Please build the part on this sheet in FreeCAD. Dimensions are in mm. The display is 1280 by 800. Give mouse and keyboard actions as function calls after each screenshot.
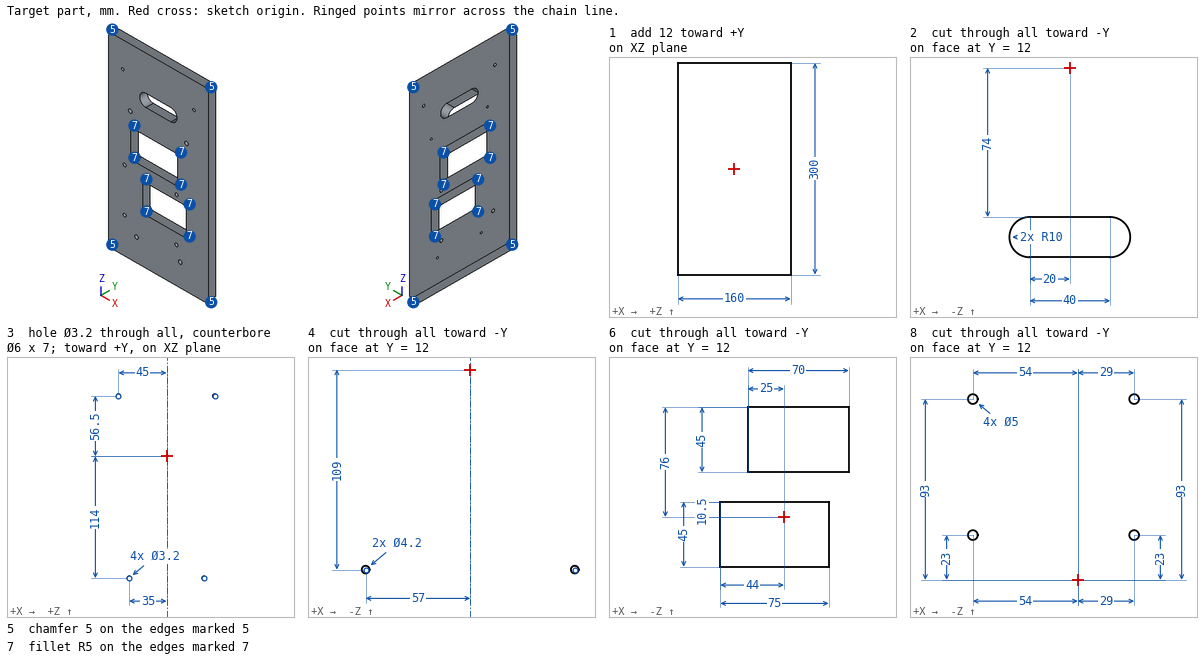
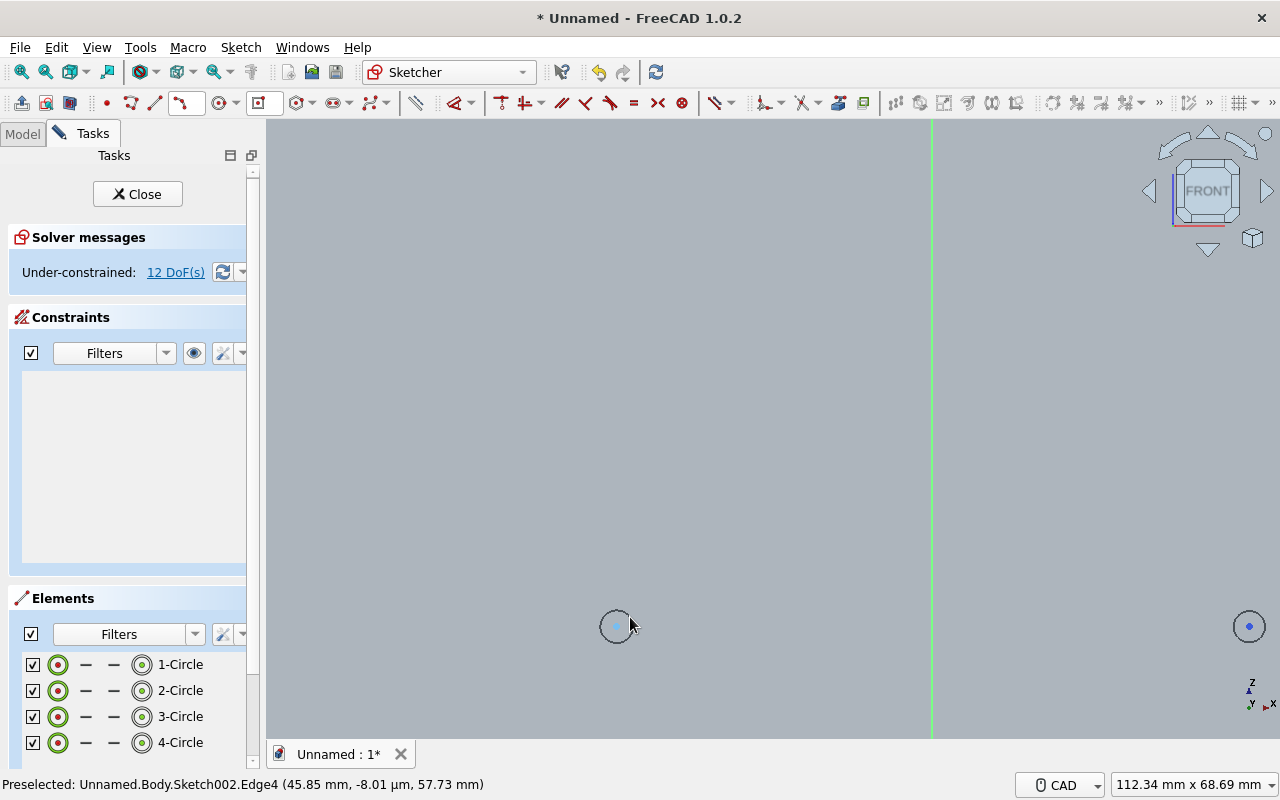
click(628, 615)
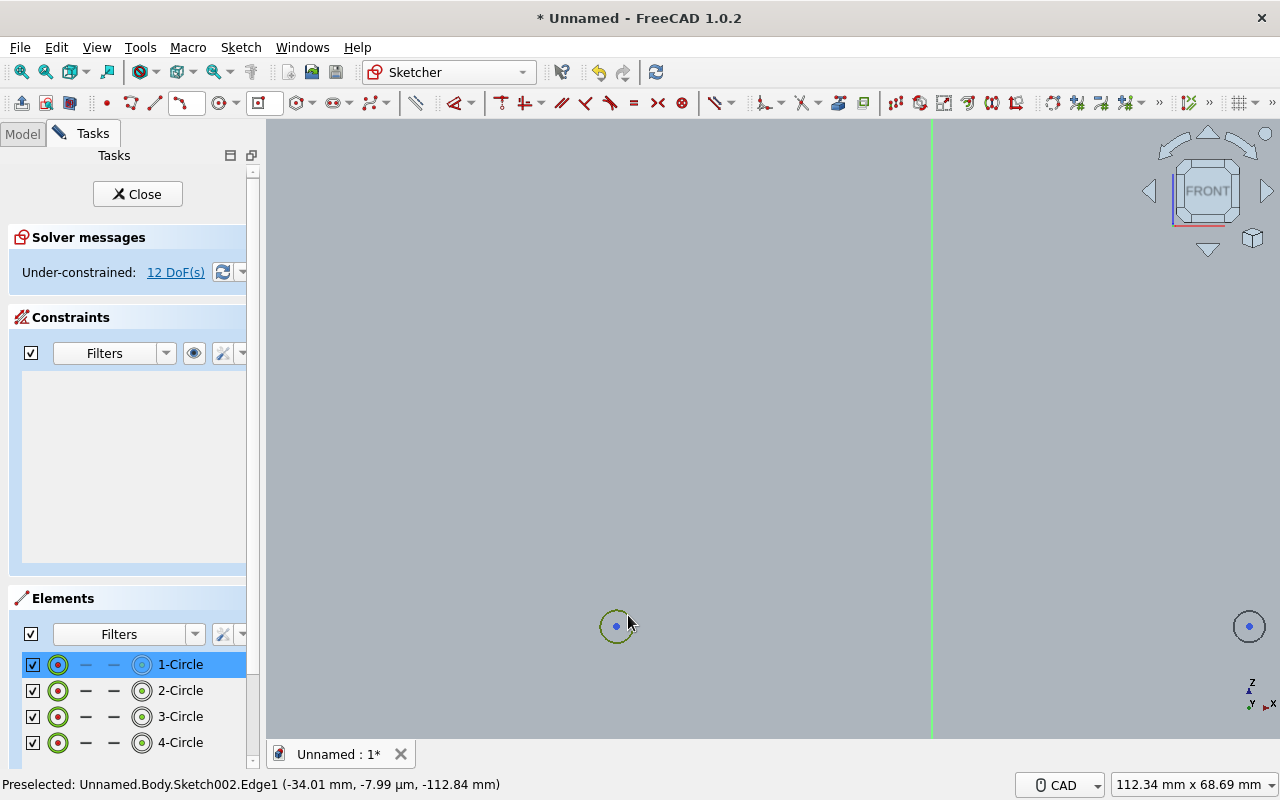
scroll(630, 617, down, 7)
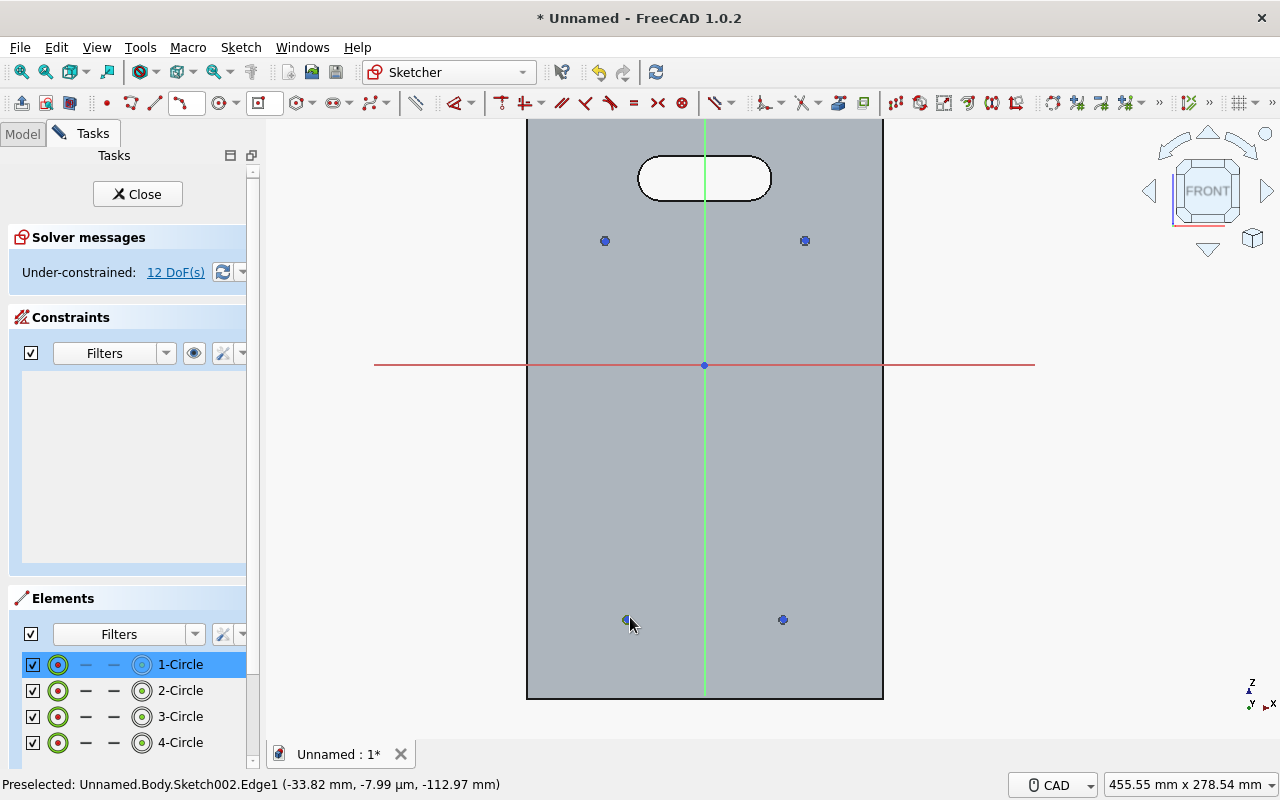
scroll(786, 617, up, 7)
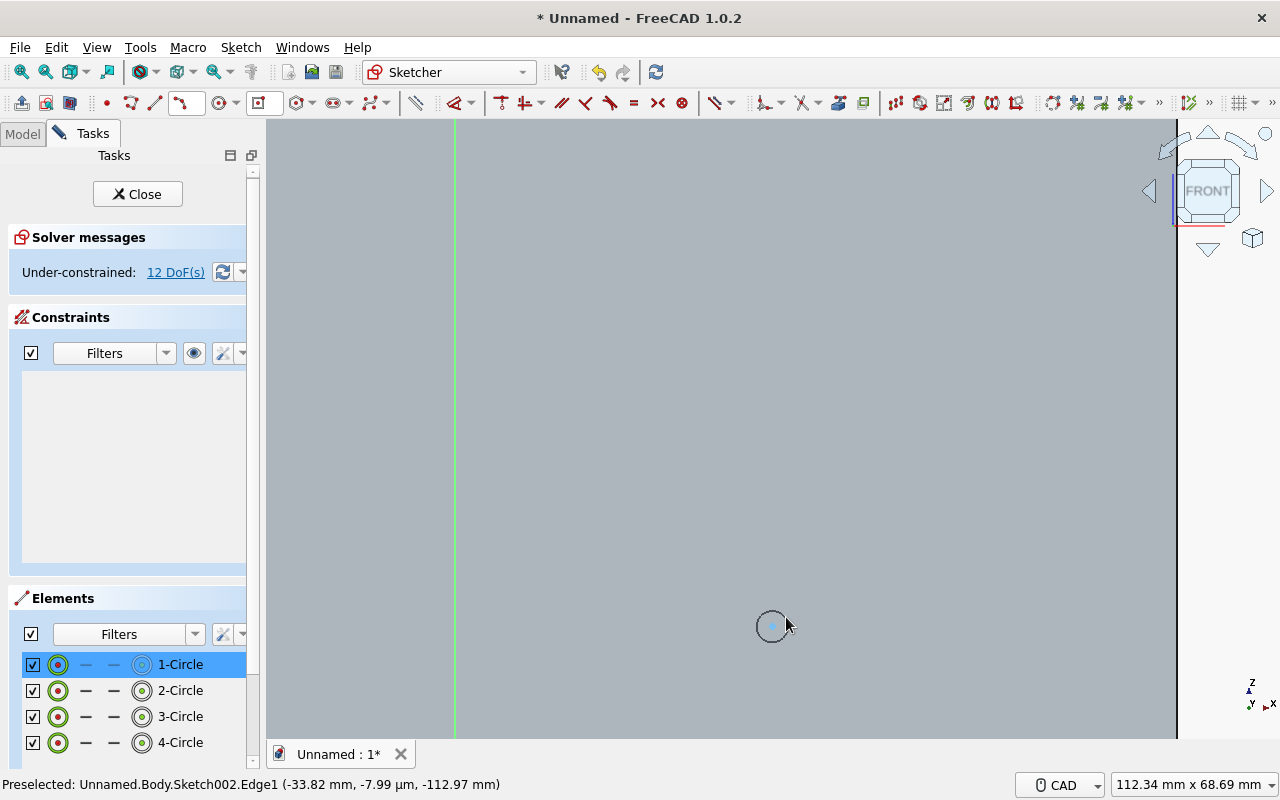
click(783, 616)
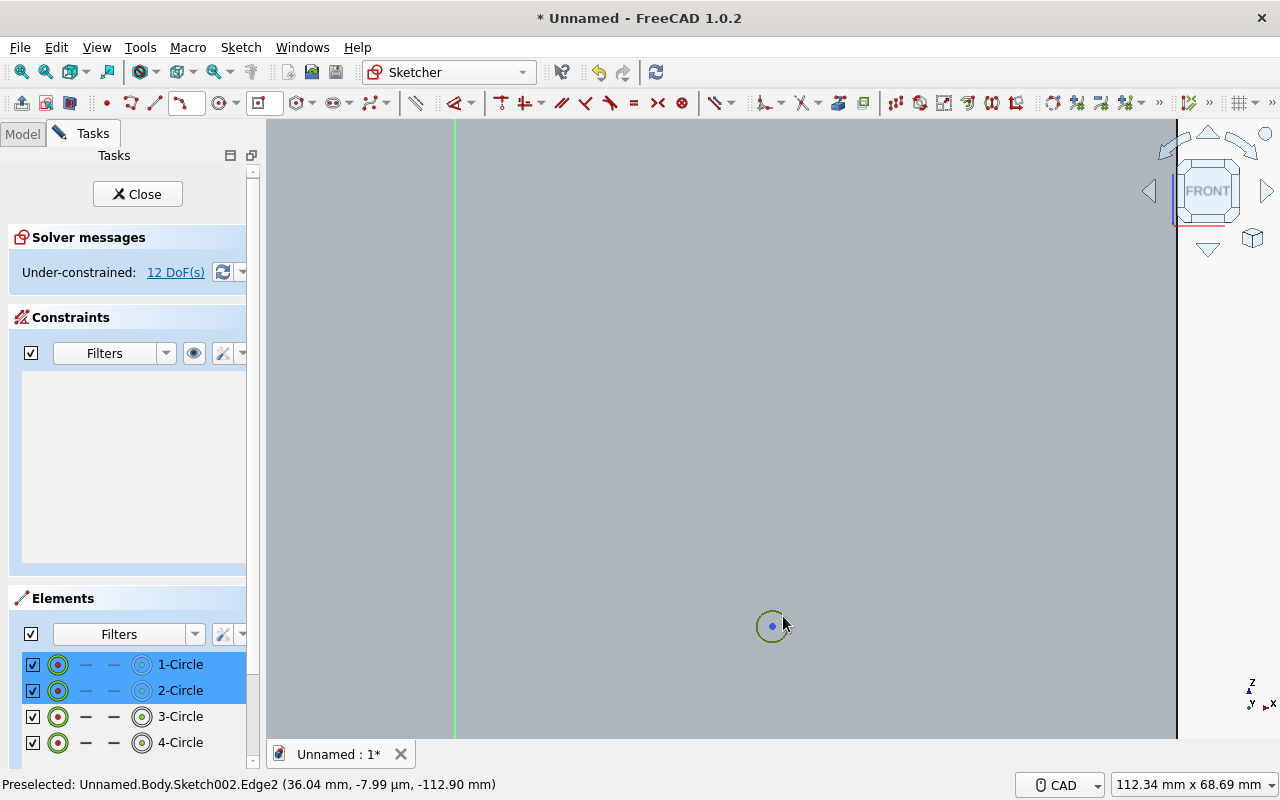
scroll(786, 617, down, 7)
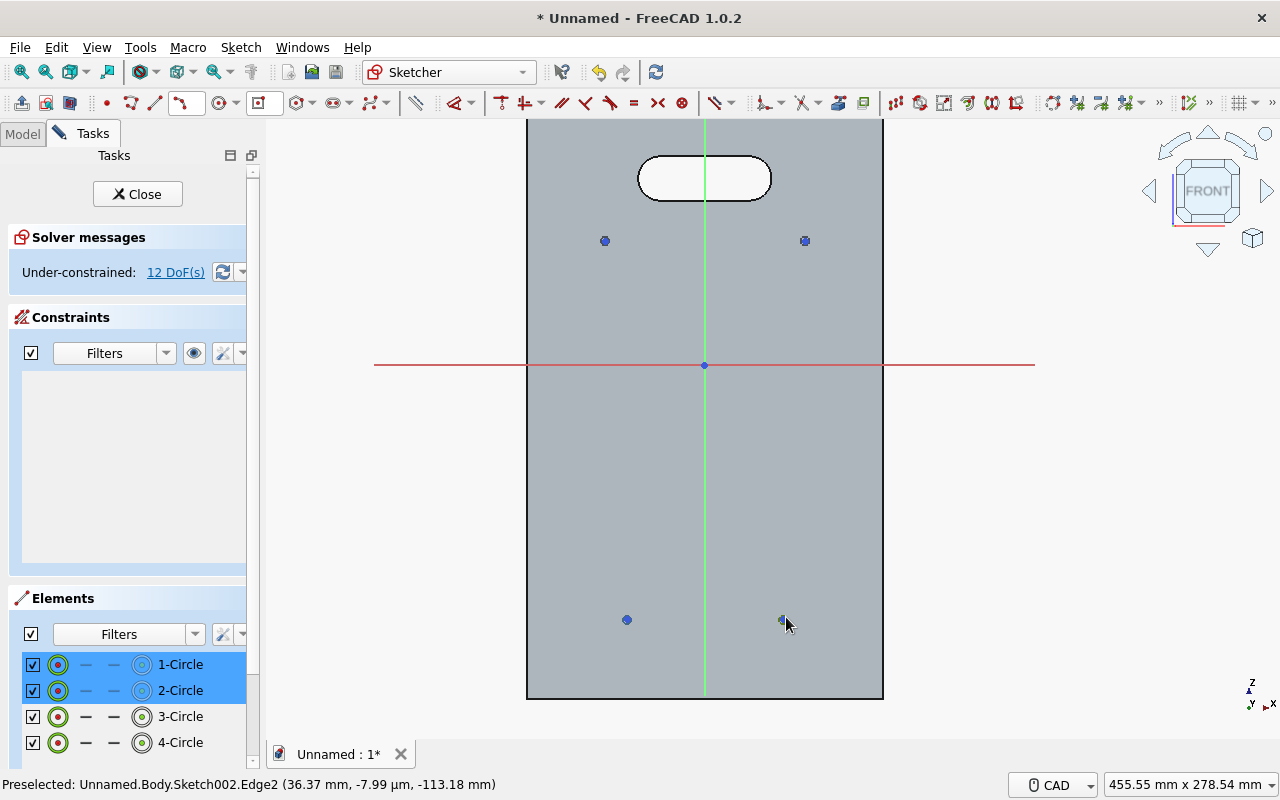
scroll(608, 238, up, 6)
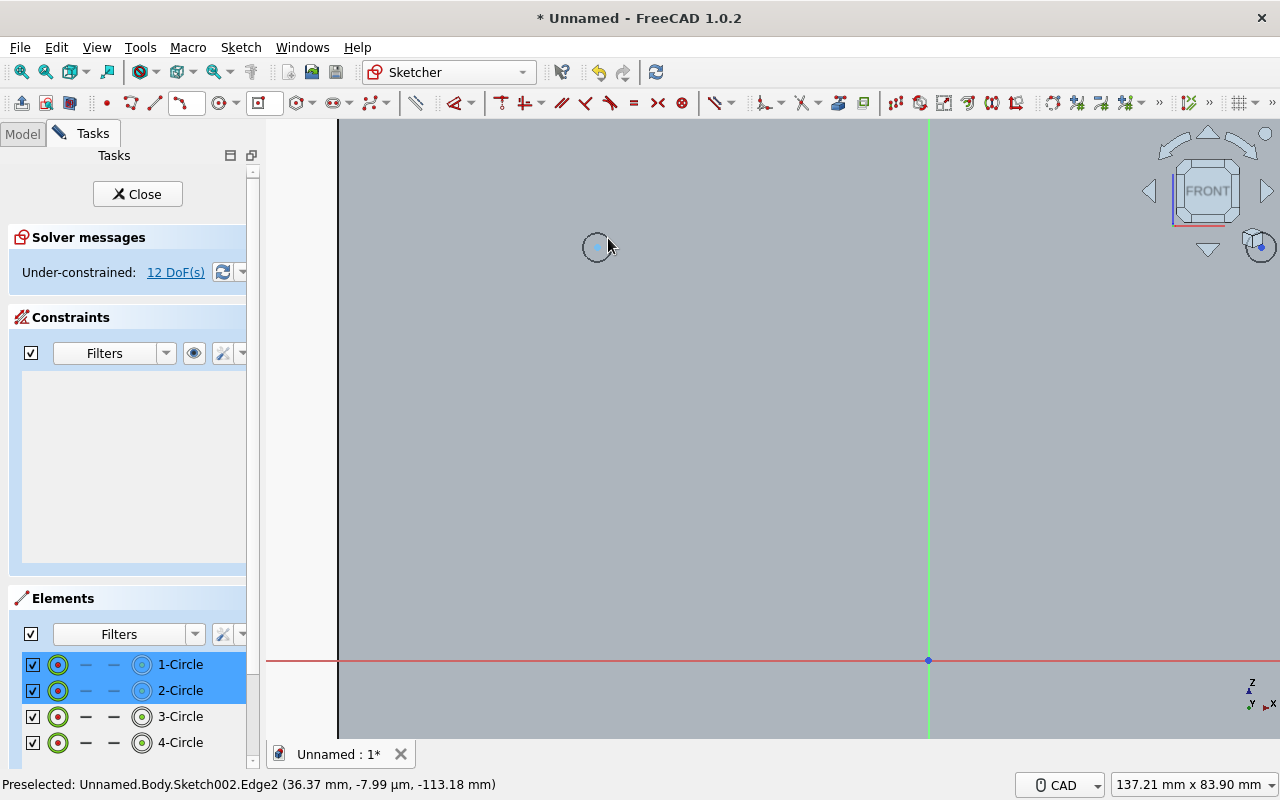
click(607, 237)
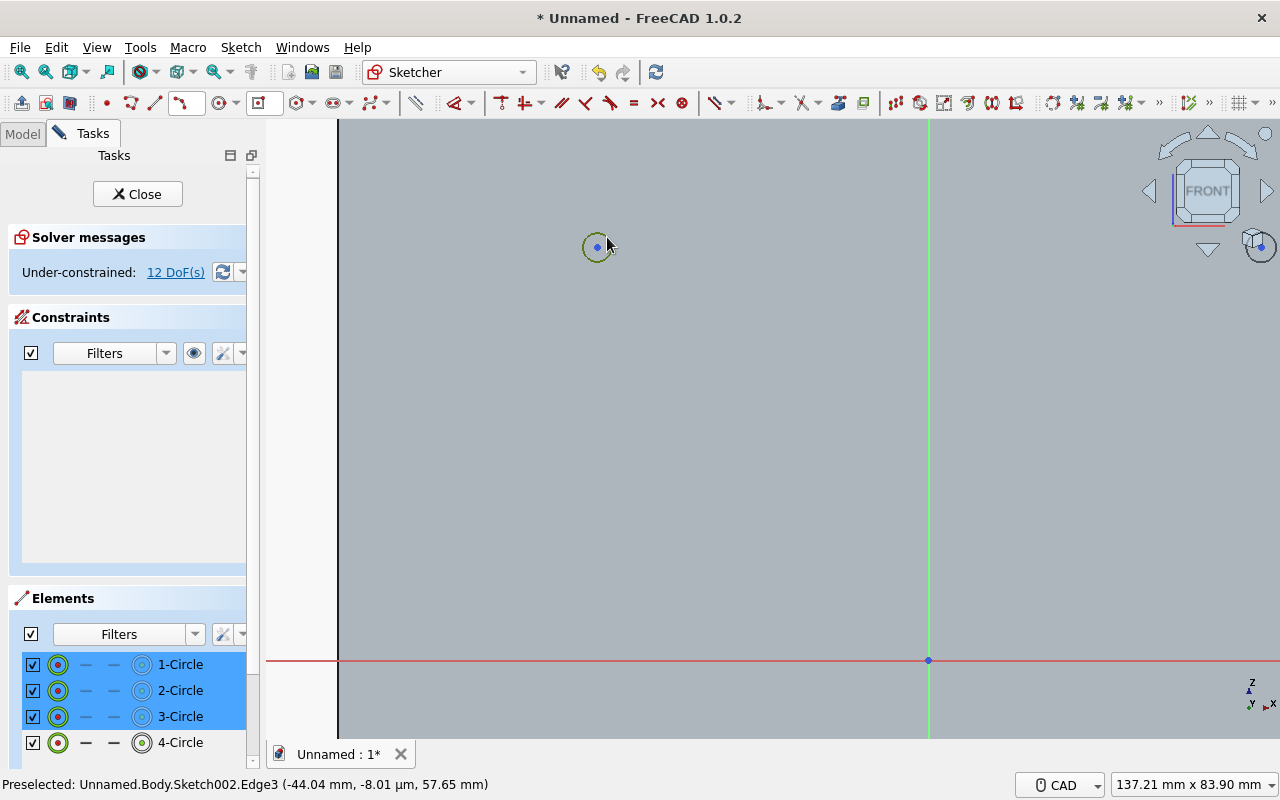
scroll(608, 238, down, 6)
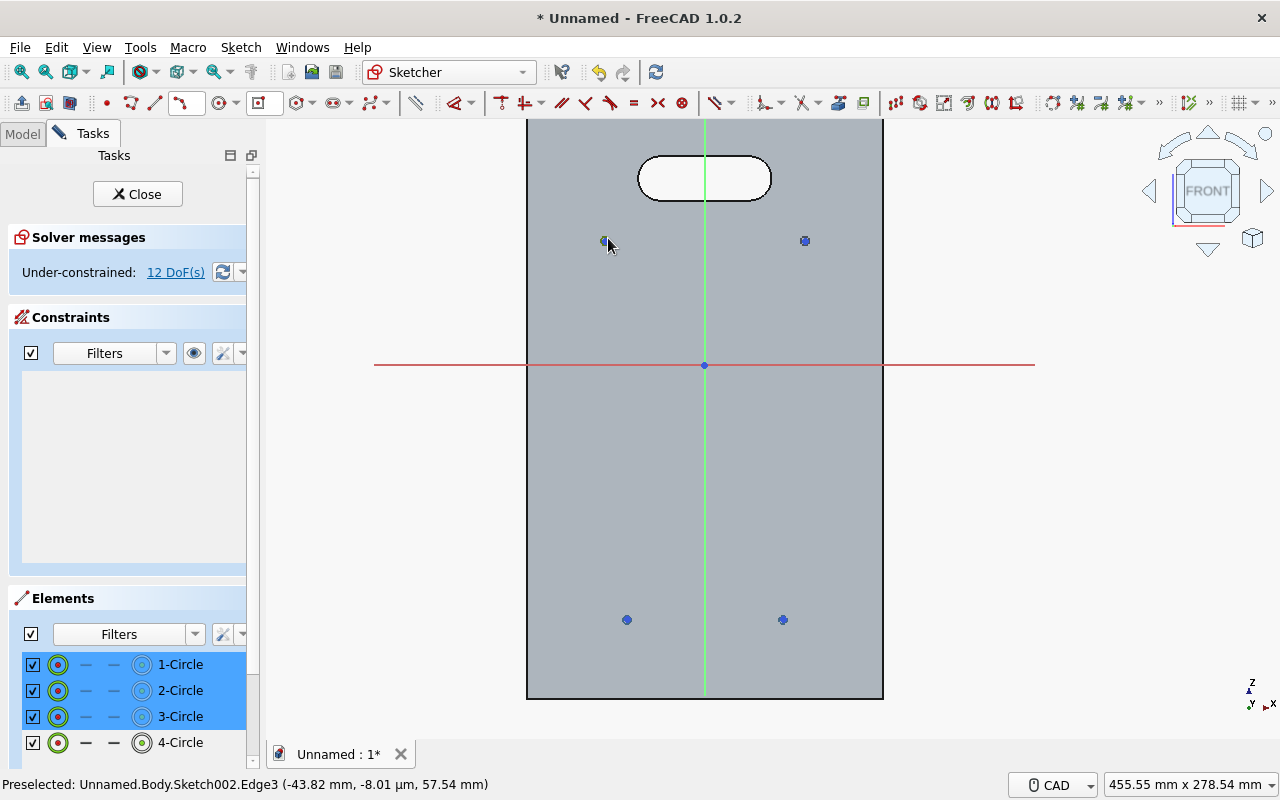
scroll(808, 238, up, 6)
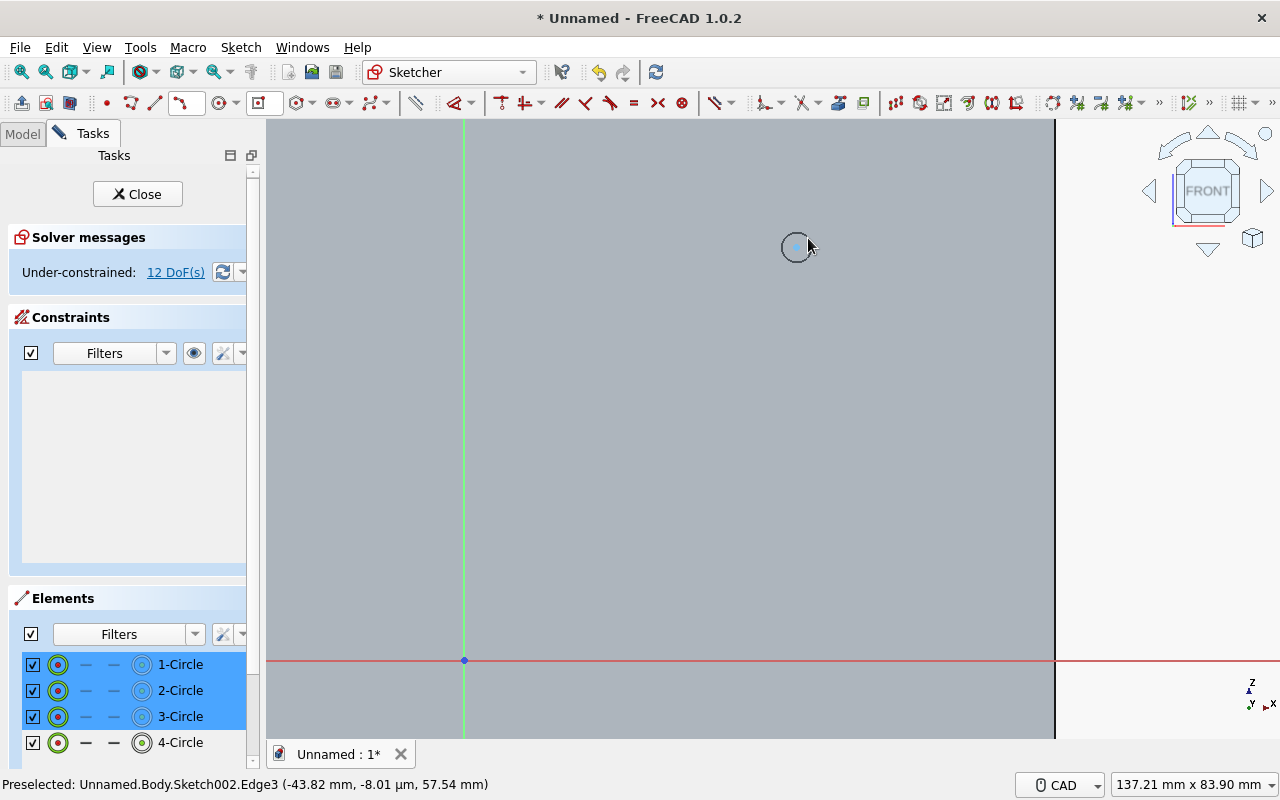
click(807, 237)